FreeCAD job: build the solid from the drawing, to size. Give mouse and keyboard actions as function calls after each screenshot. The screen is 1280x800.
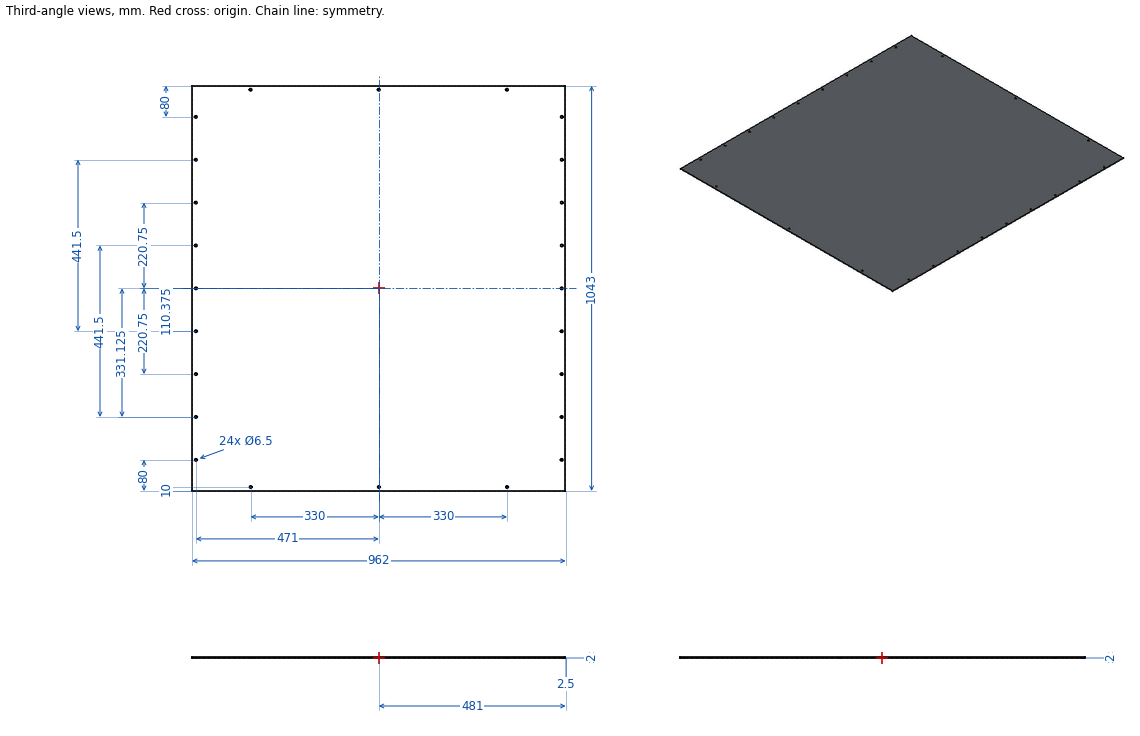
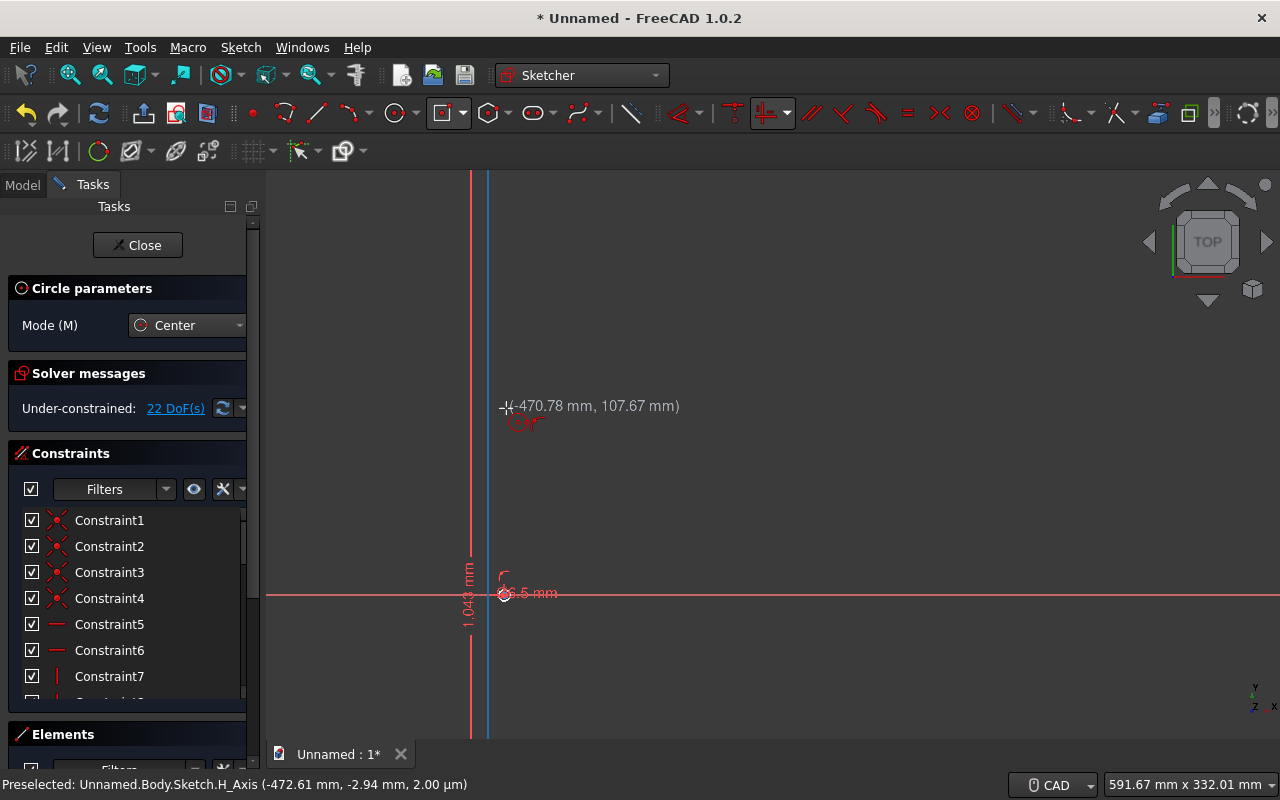
click(505, 406)
move(509, 402)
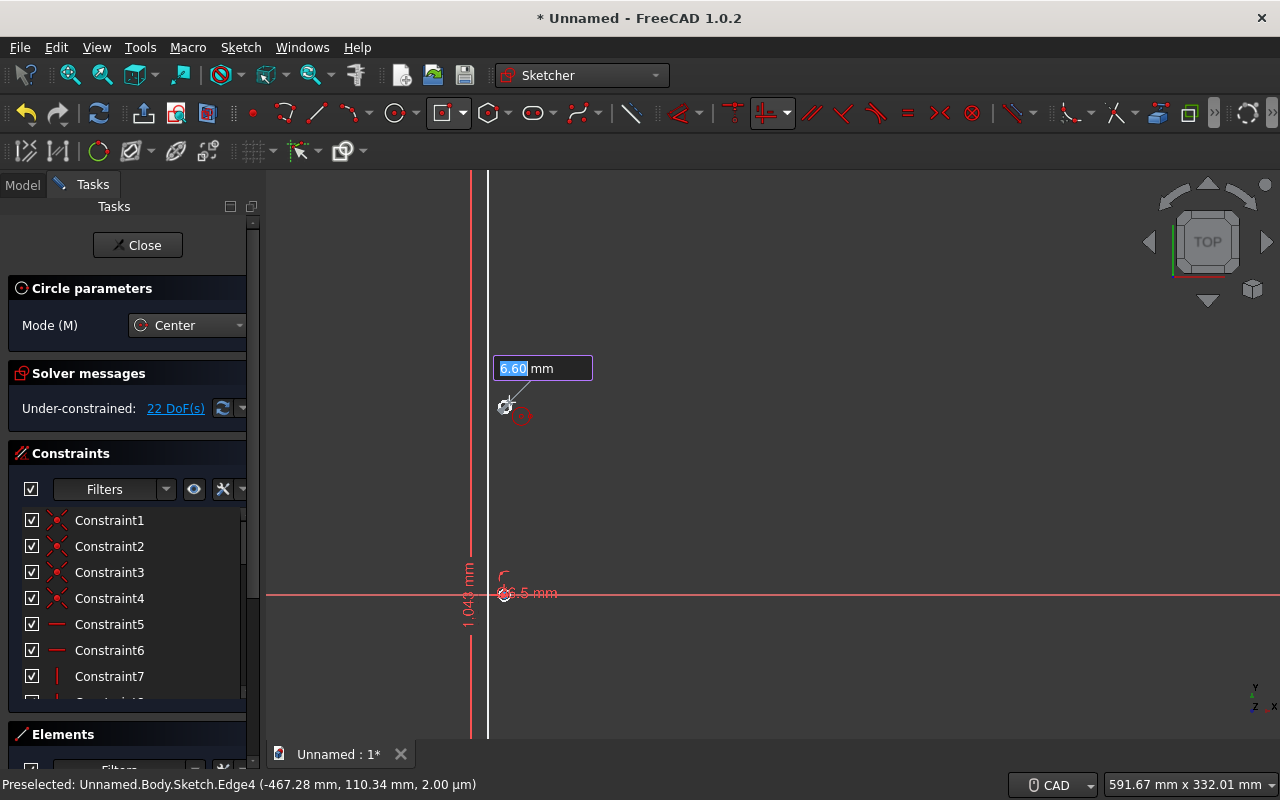
text(6.5)
key(Return)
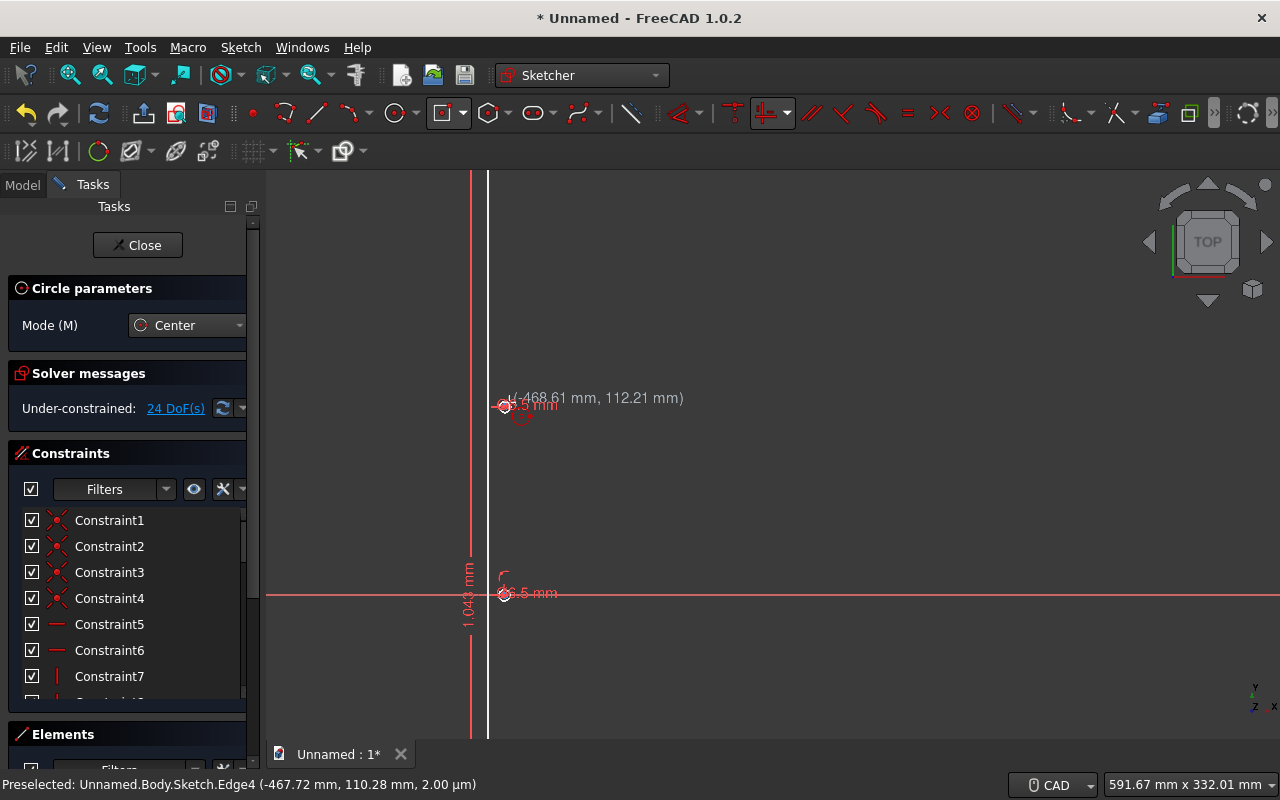
scroll(505, 217, up, 8)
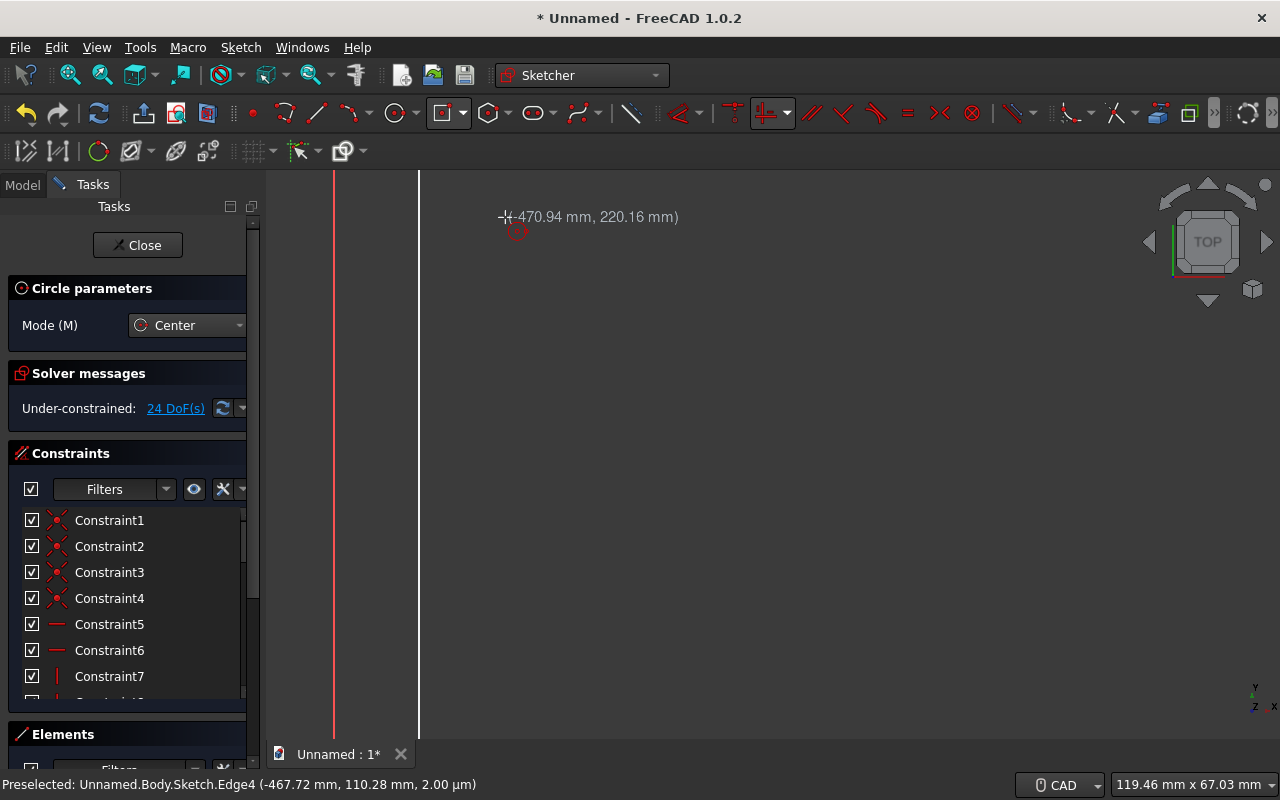
scroll(506, 369, down, 15)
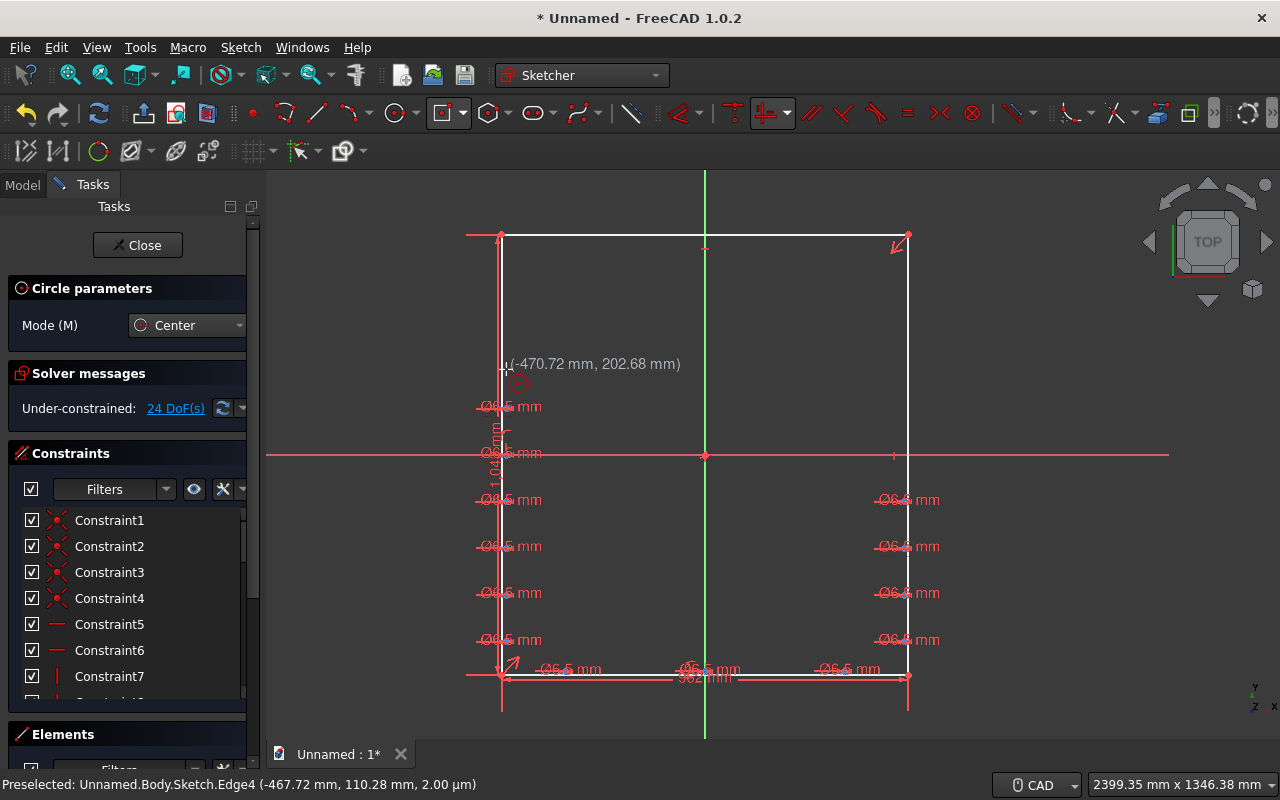
scroll(506, 362, up, 7)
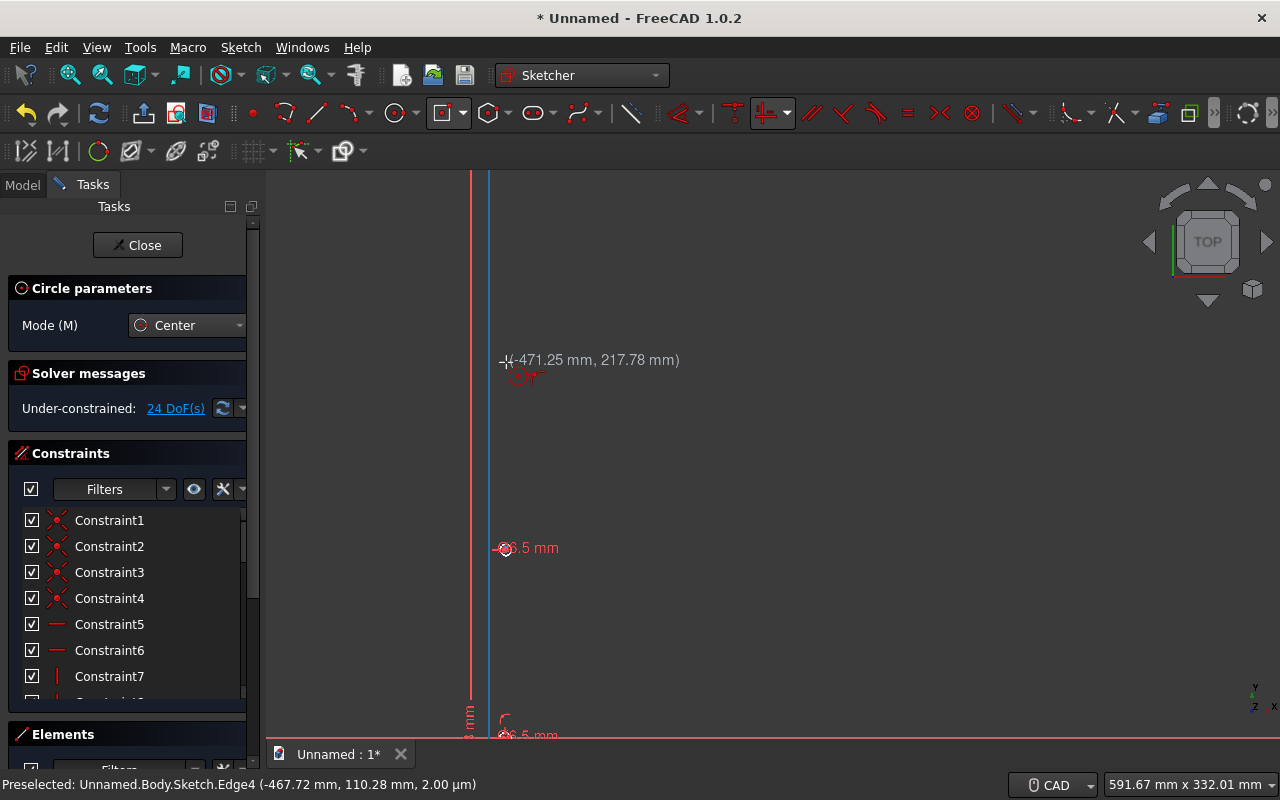
click(506, 360)
move(510, 356)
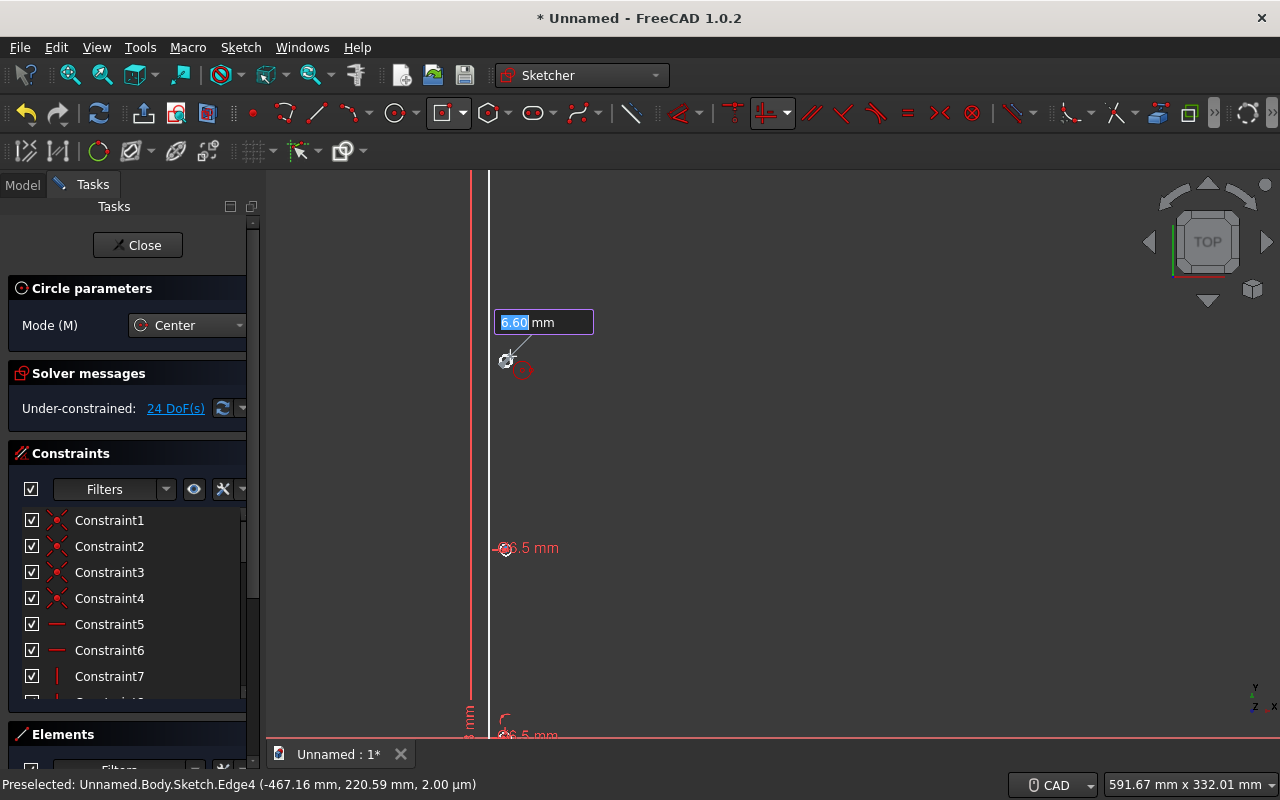
text(6.5)
key(Return)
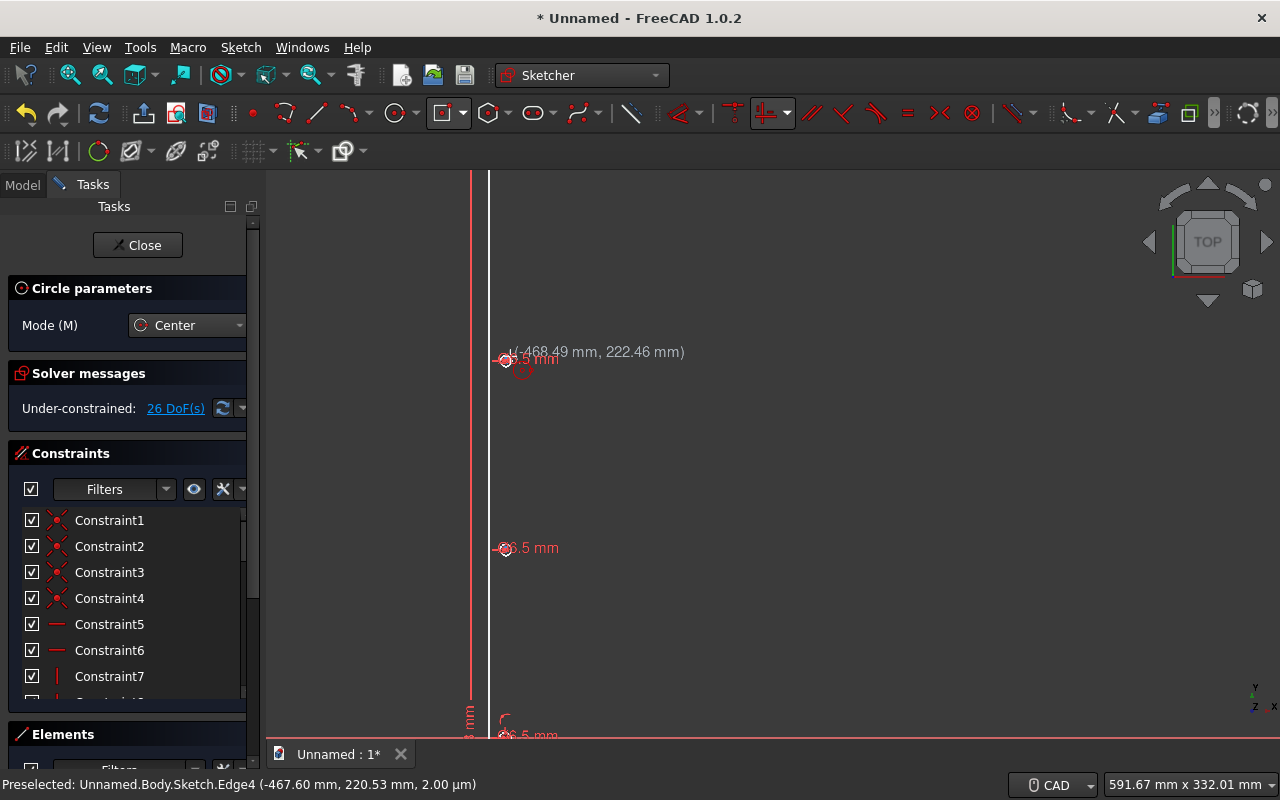
scroll(551, 383, down, 8)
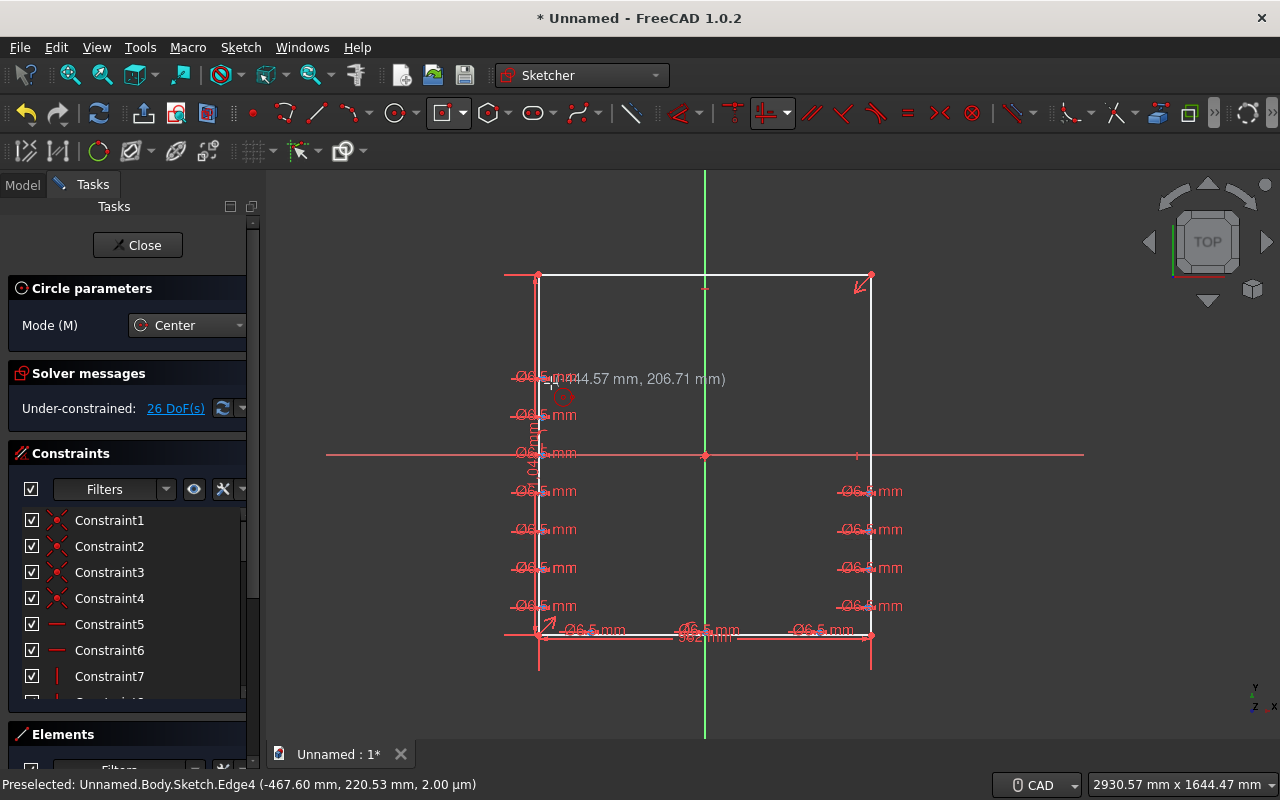
scroll(542, 340, up, 16)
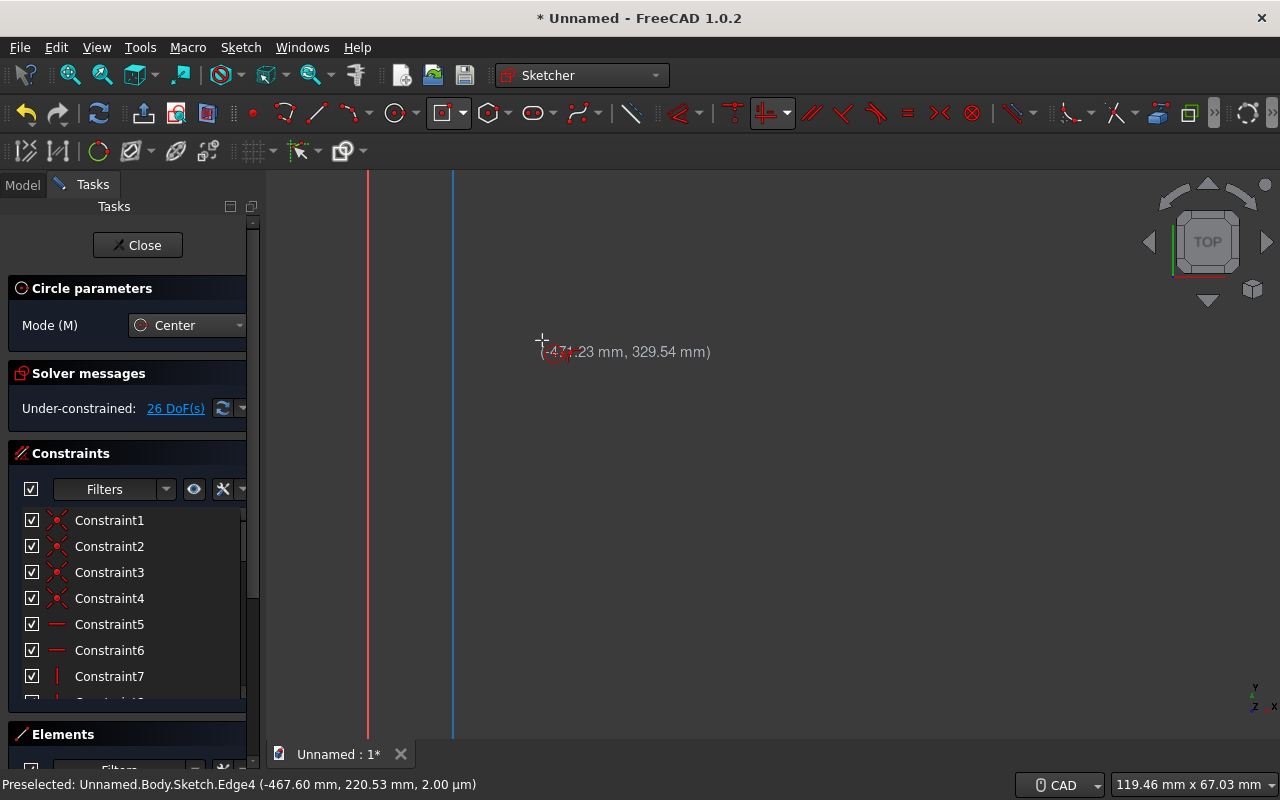
scroll(504, 313, down, 15)